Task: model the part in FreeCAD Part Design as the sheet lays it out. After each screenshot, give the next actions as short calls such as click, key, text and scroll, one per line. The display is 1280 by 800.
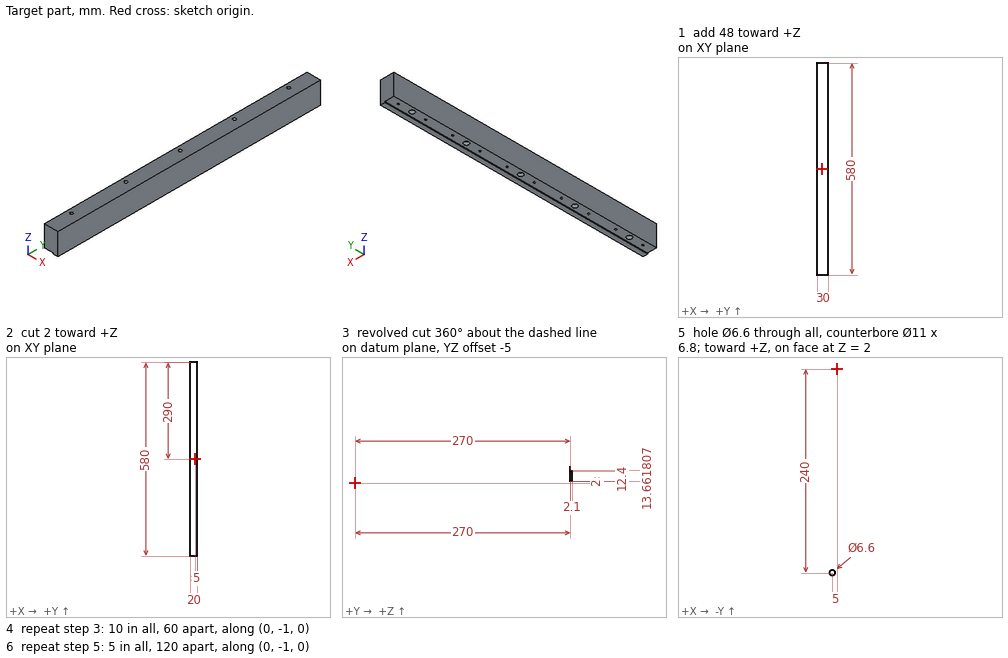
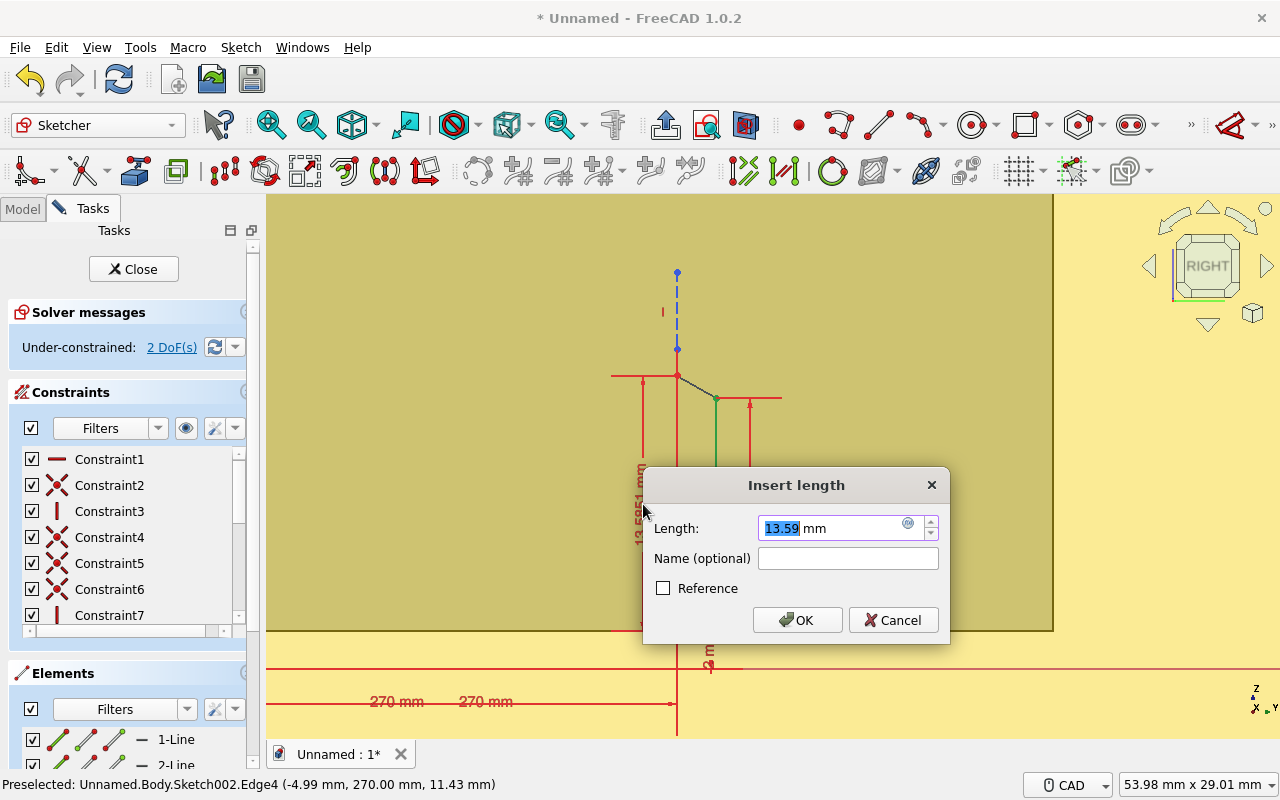
text(13.661807)
key(Return)
key(Escape)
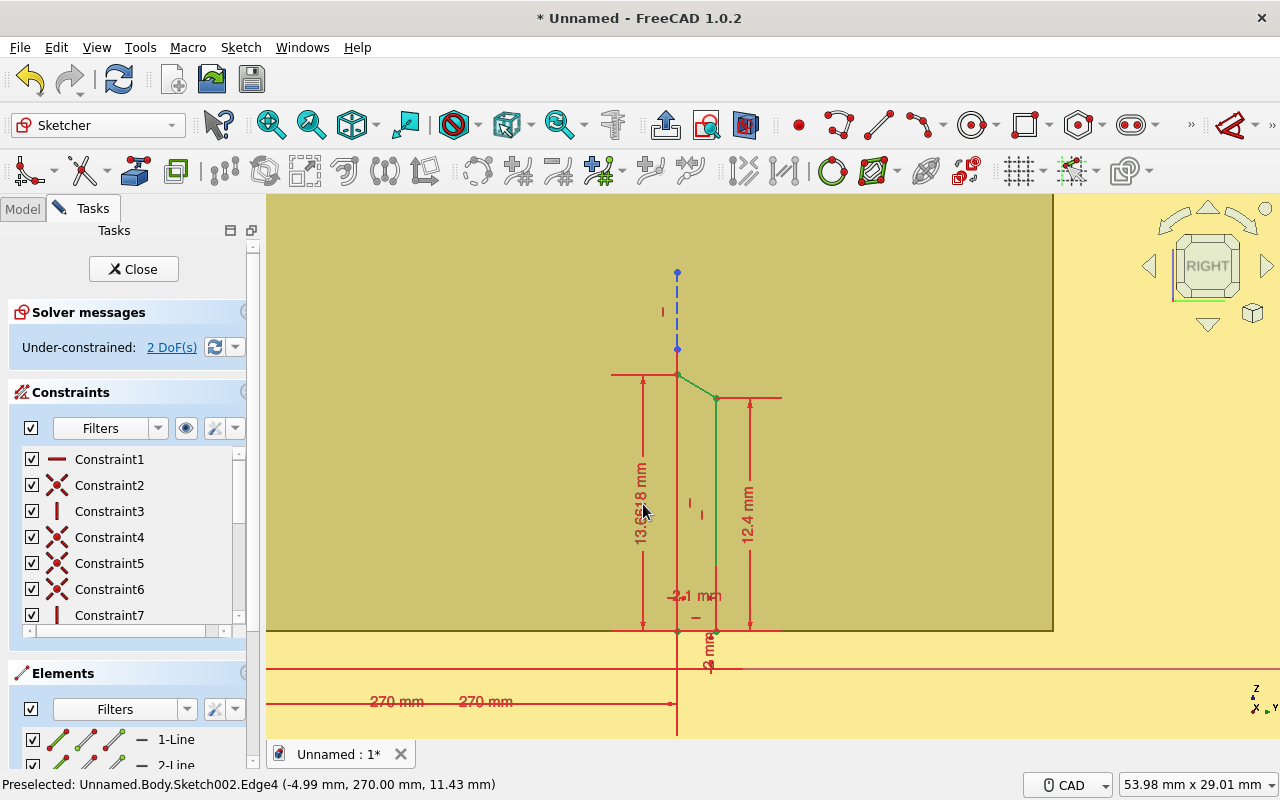
click(134, 269)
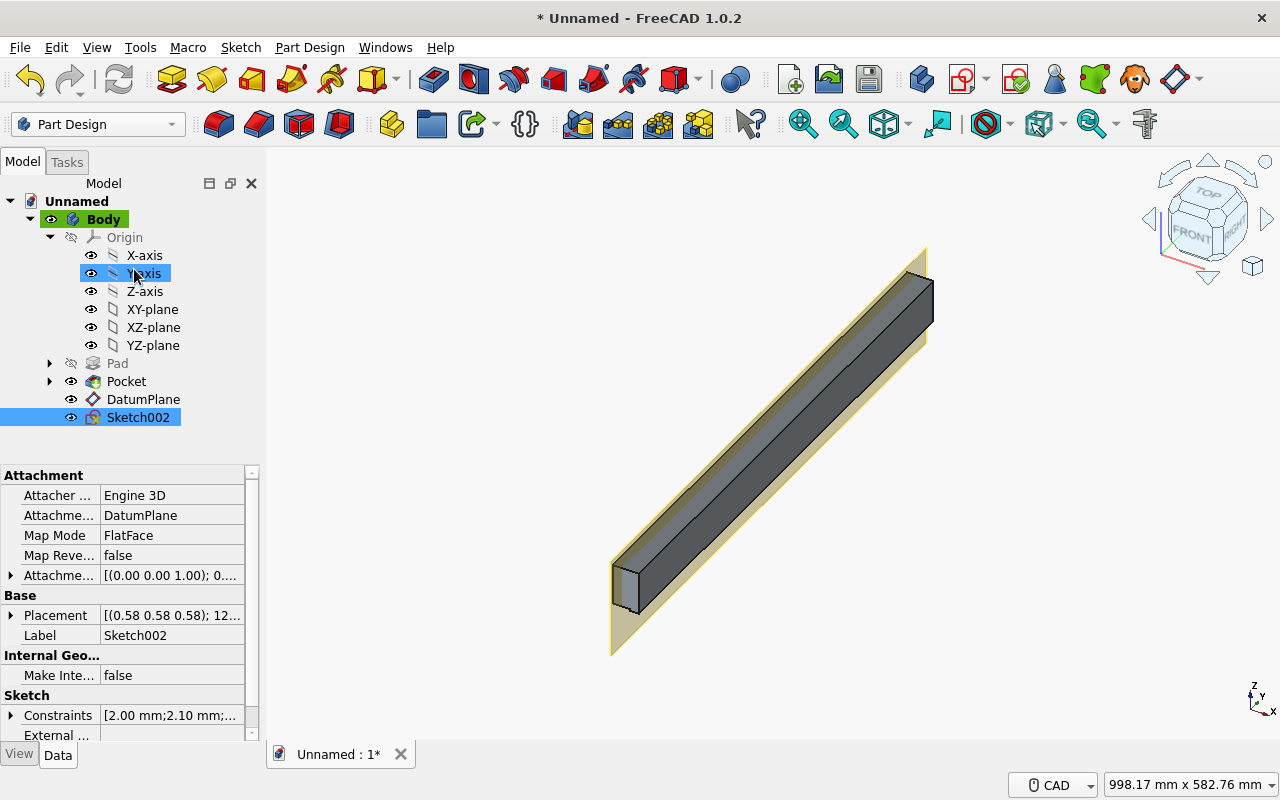
click(514, 80)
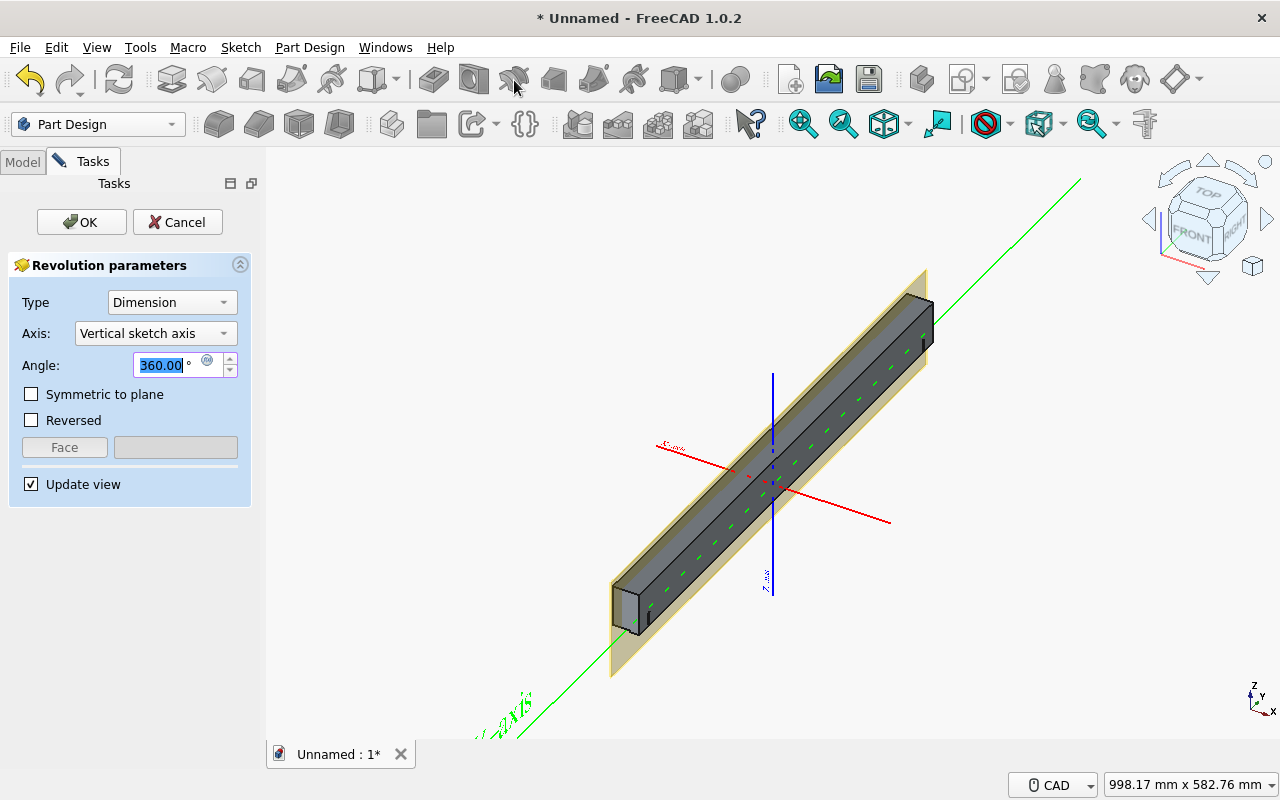
click(156, 334)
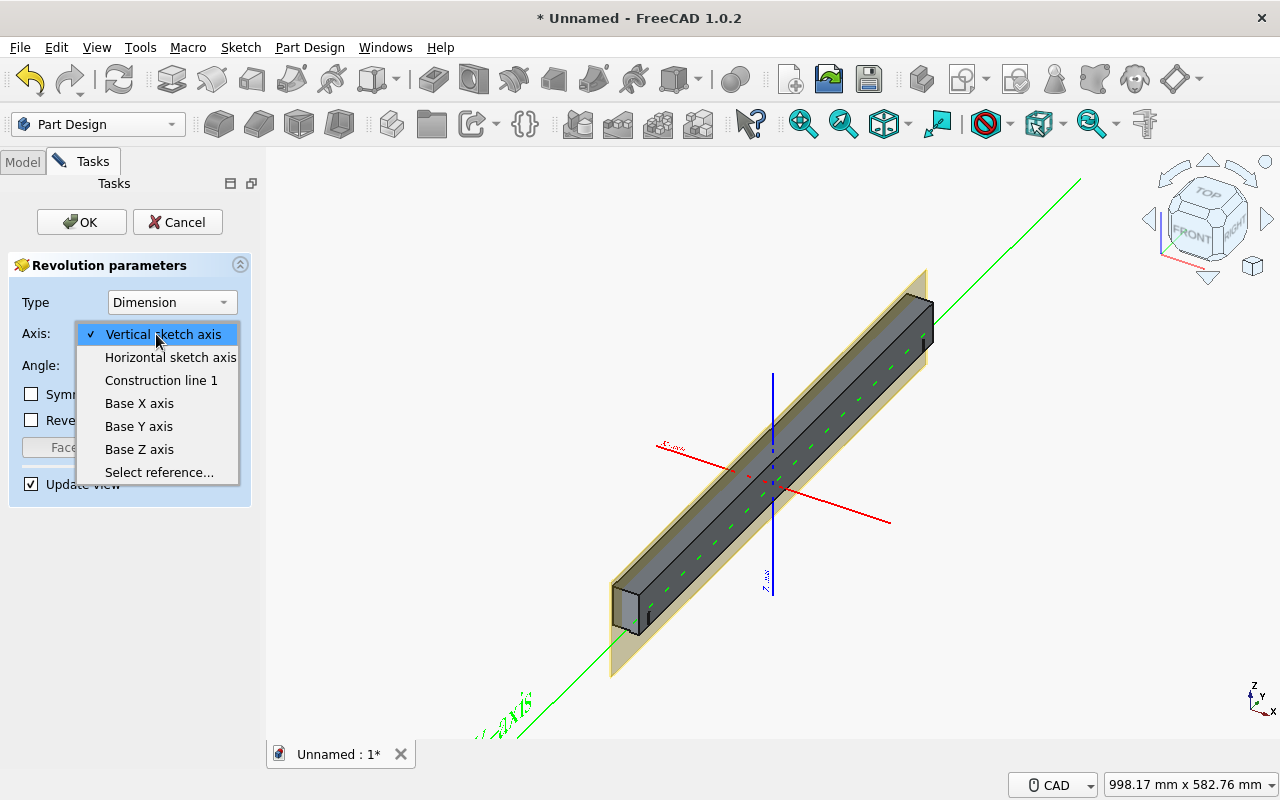
click(156, 380)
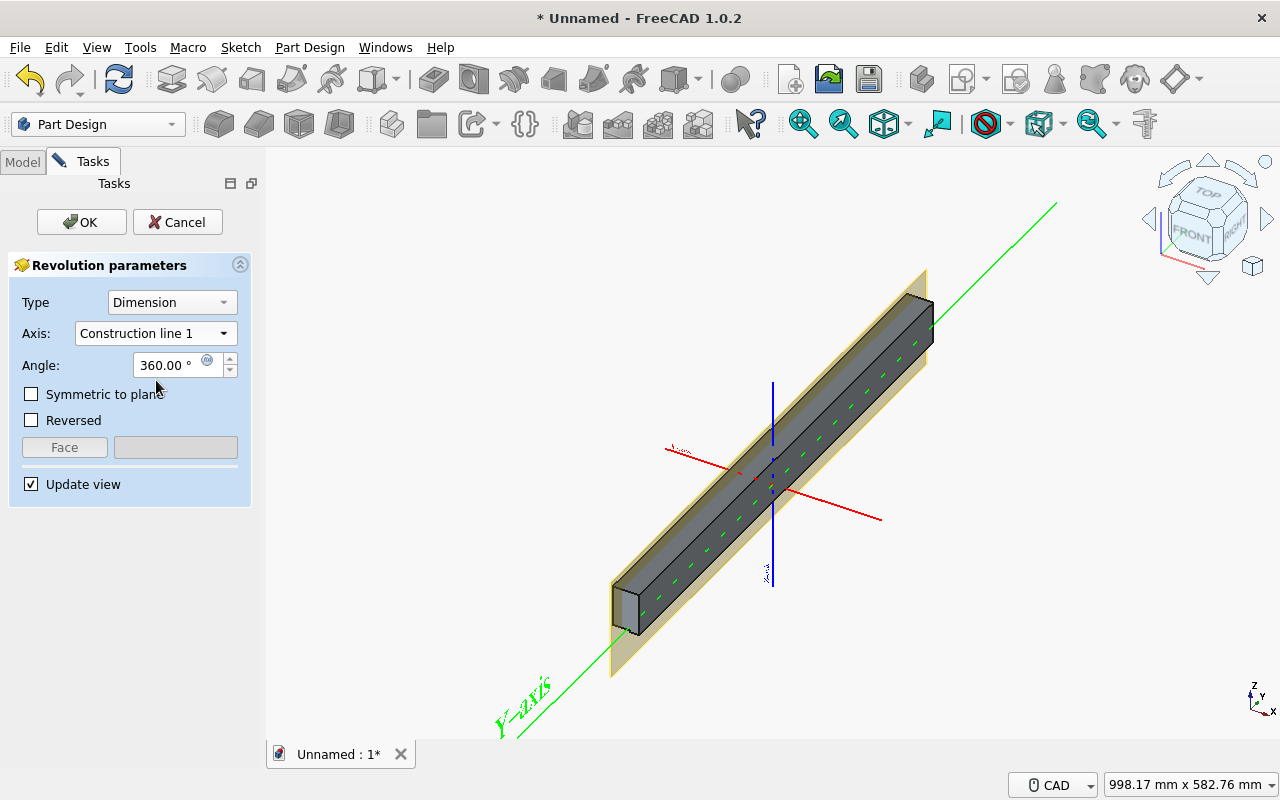
click(82, 222)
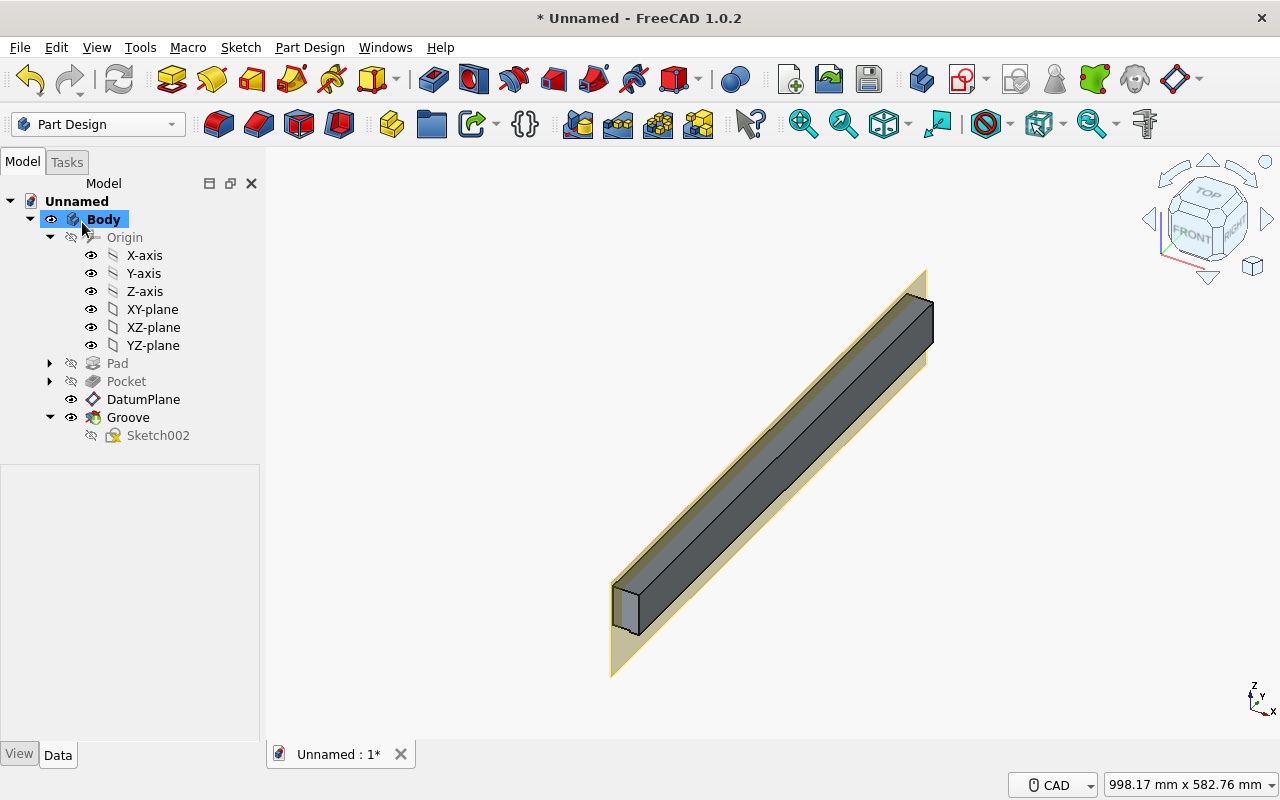
click(116, 399)
key(space)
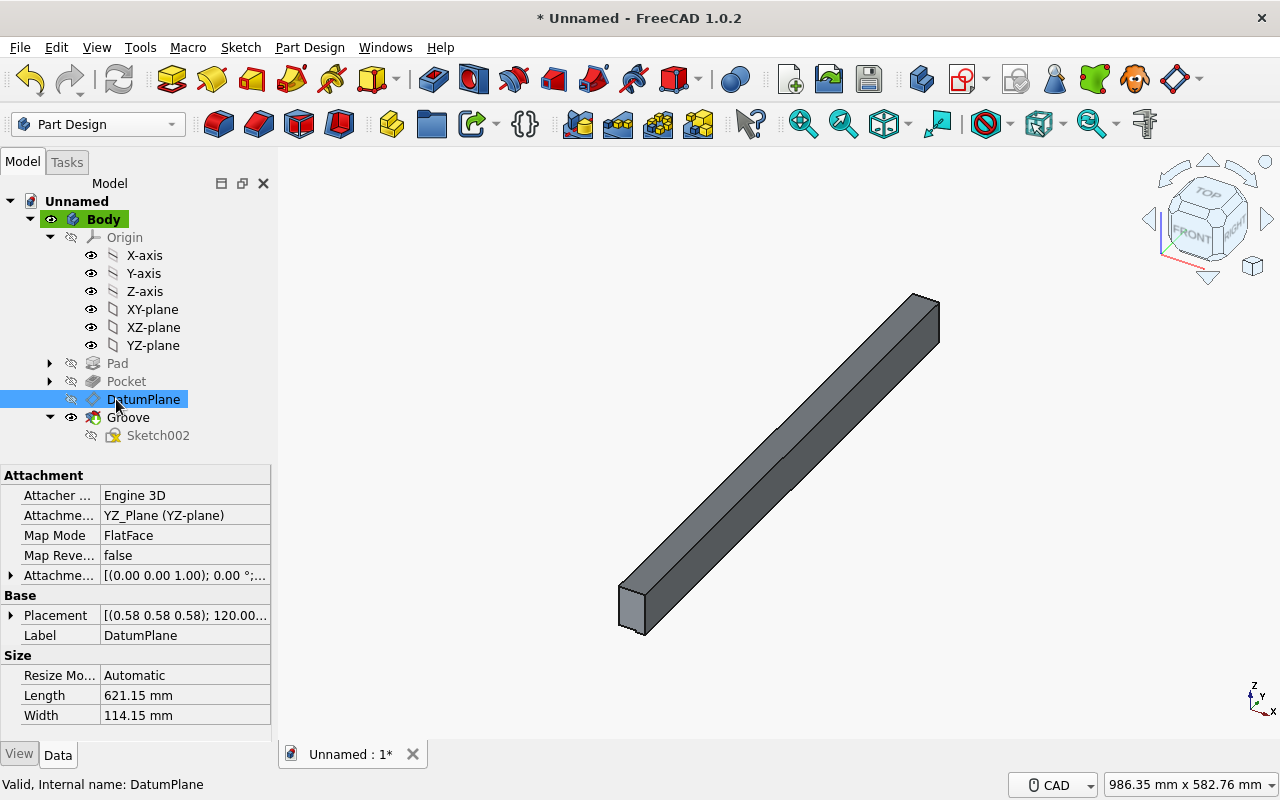
click(116, 417)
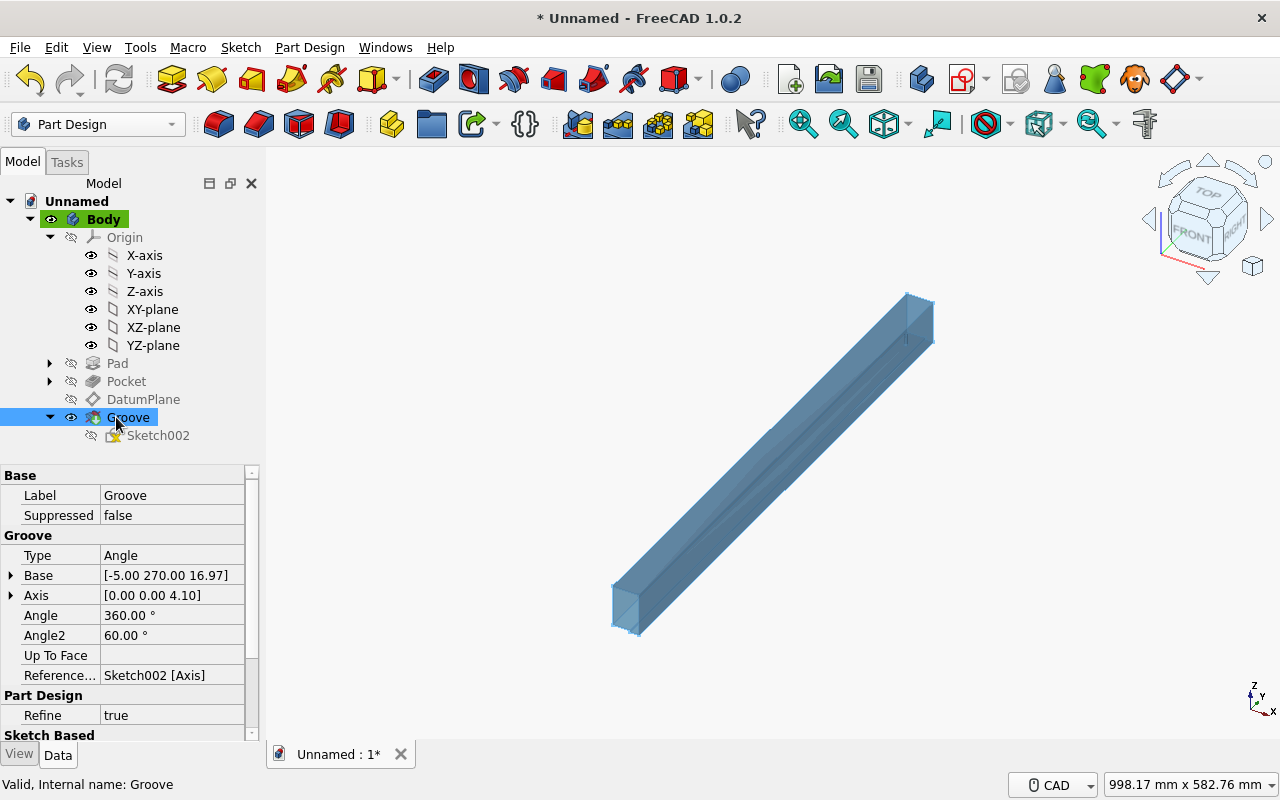
click(618, 124)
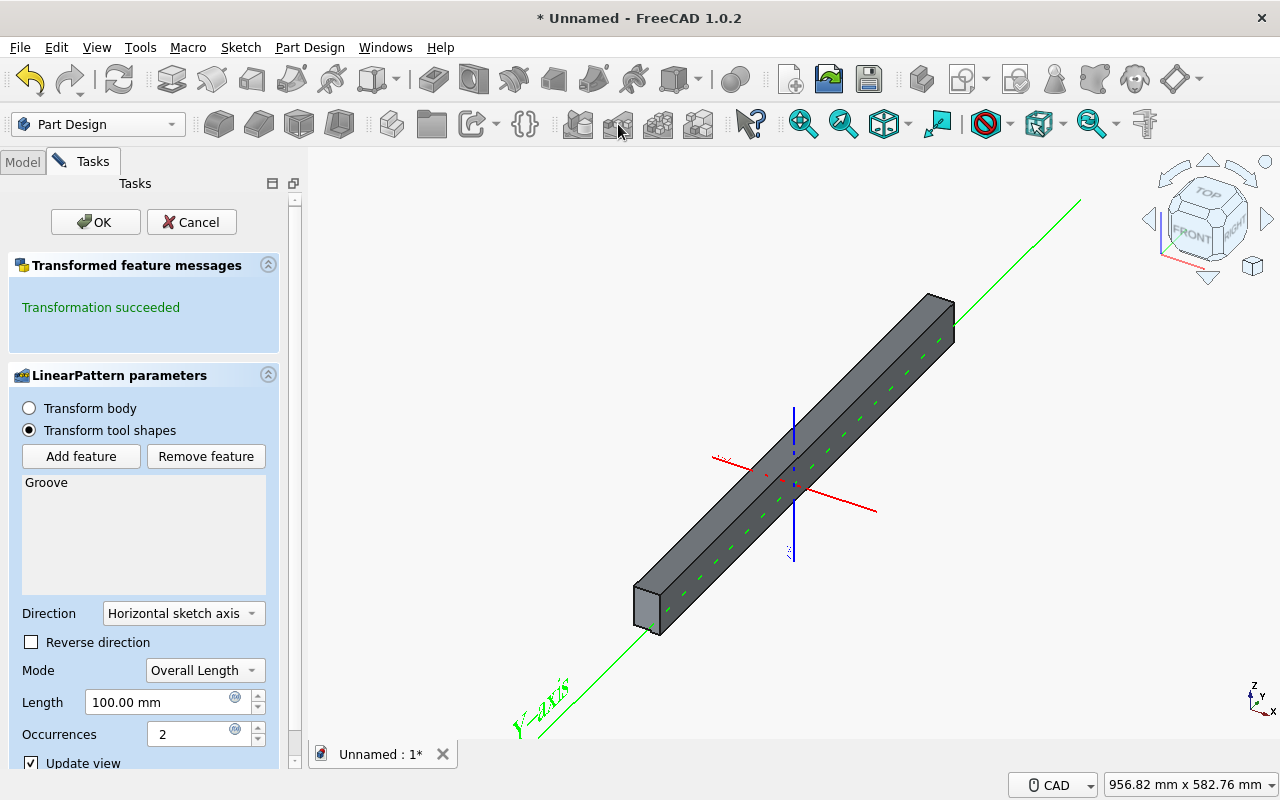
click(184, 614)